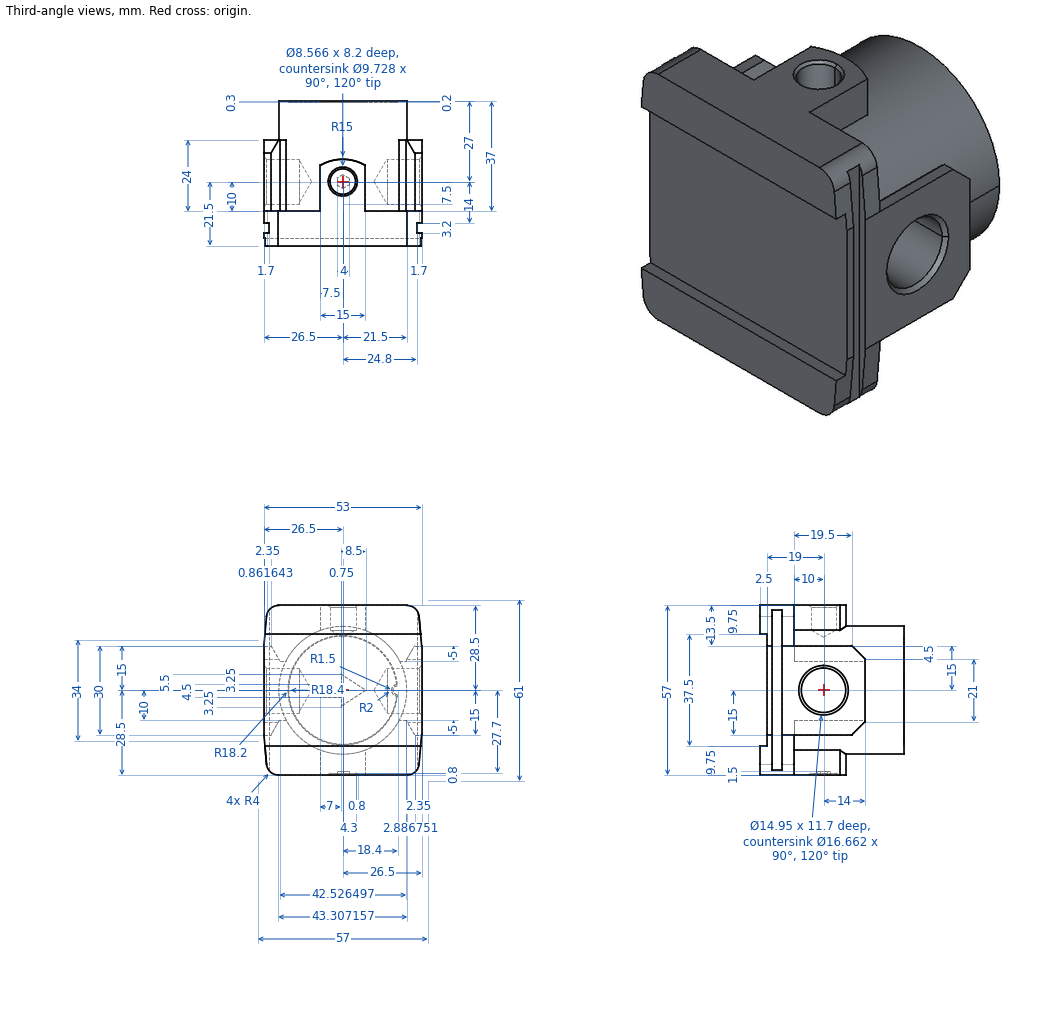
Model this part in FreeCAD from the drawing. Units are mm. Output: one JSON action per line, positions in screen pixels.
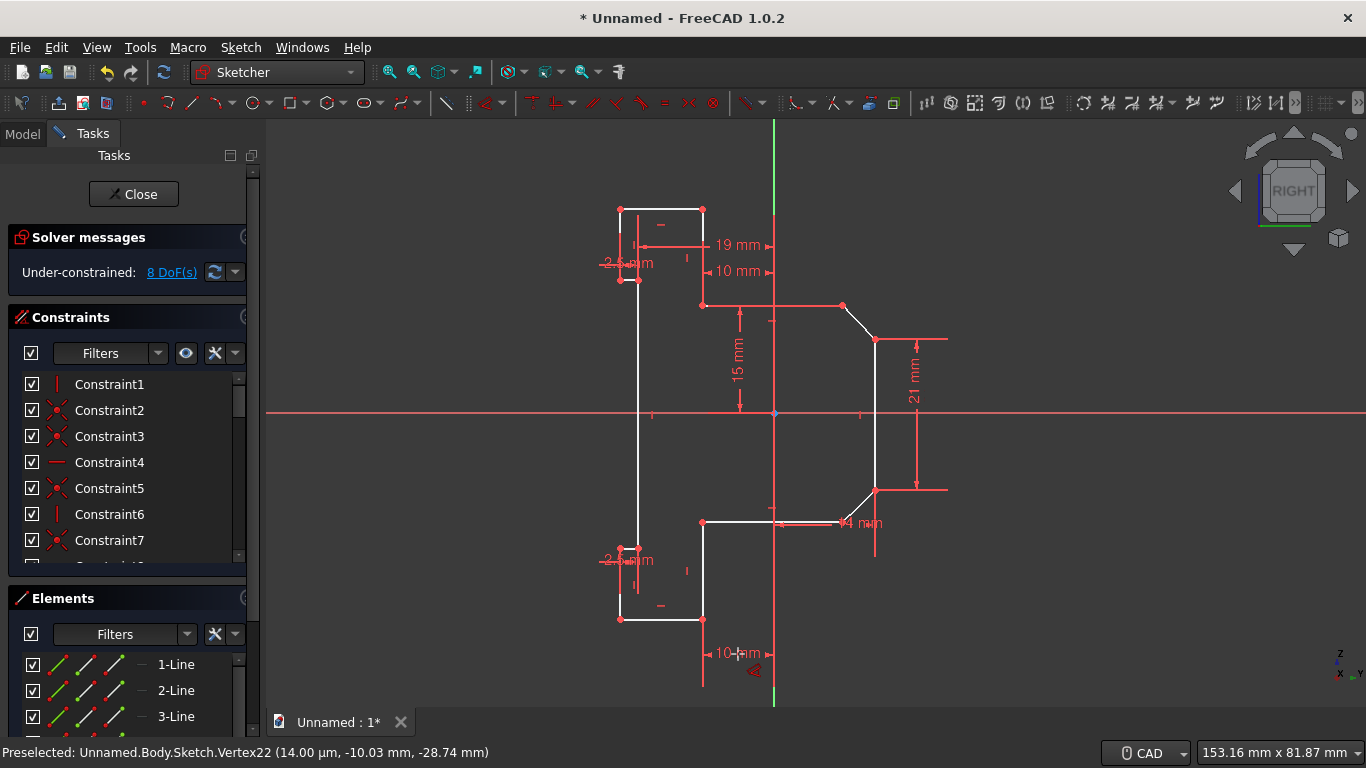
{"action": "left_click", "coordinate": [703, 522]}
{"action": "left_click", "coordinate": [669, 468]}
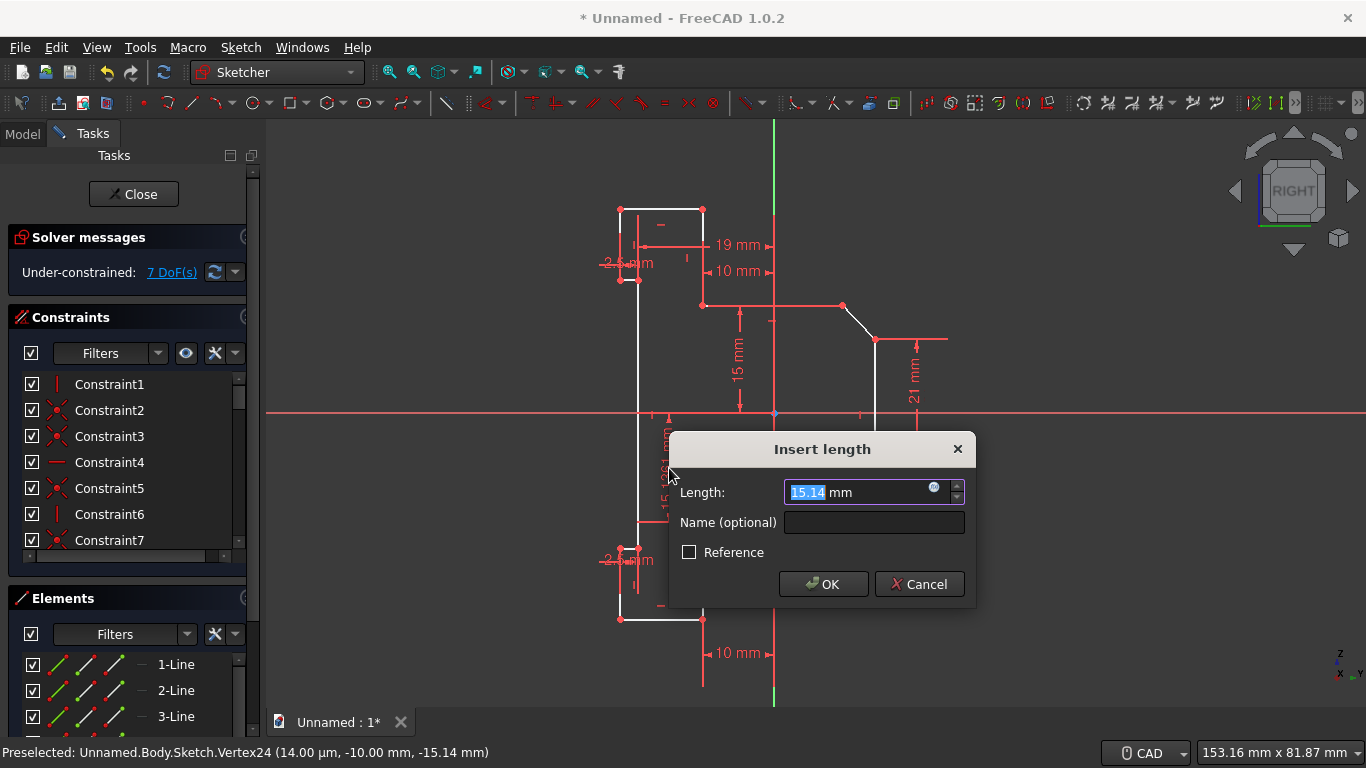
{"action": "type", "text": "15"}
{"action": "key", "text": "Return"}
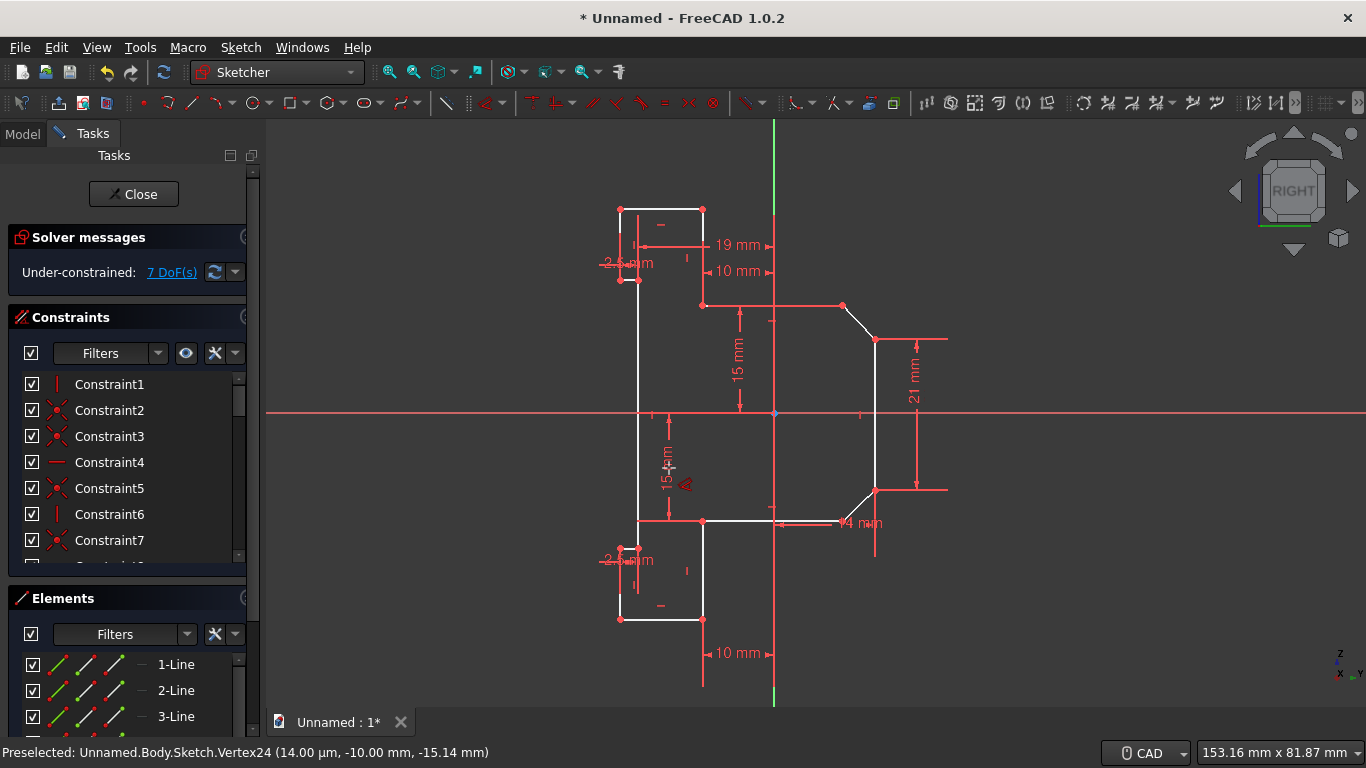
{"action": "left_click", "coordinate": [801, 306]}
{"action": "left_click", "coordinate": [822, 272]}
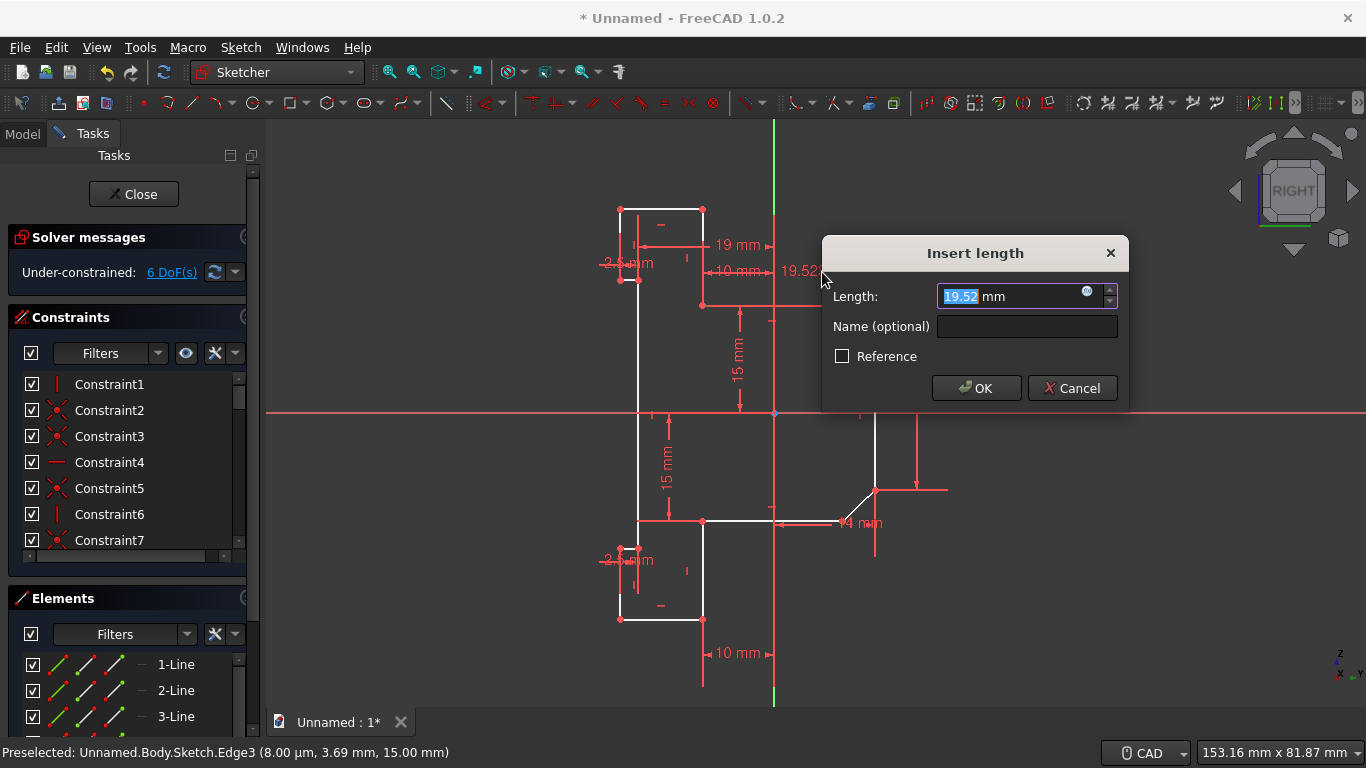
{"action": "type", "text": "19.5"}
{"action": "key", "text": "Return"}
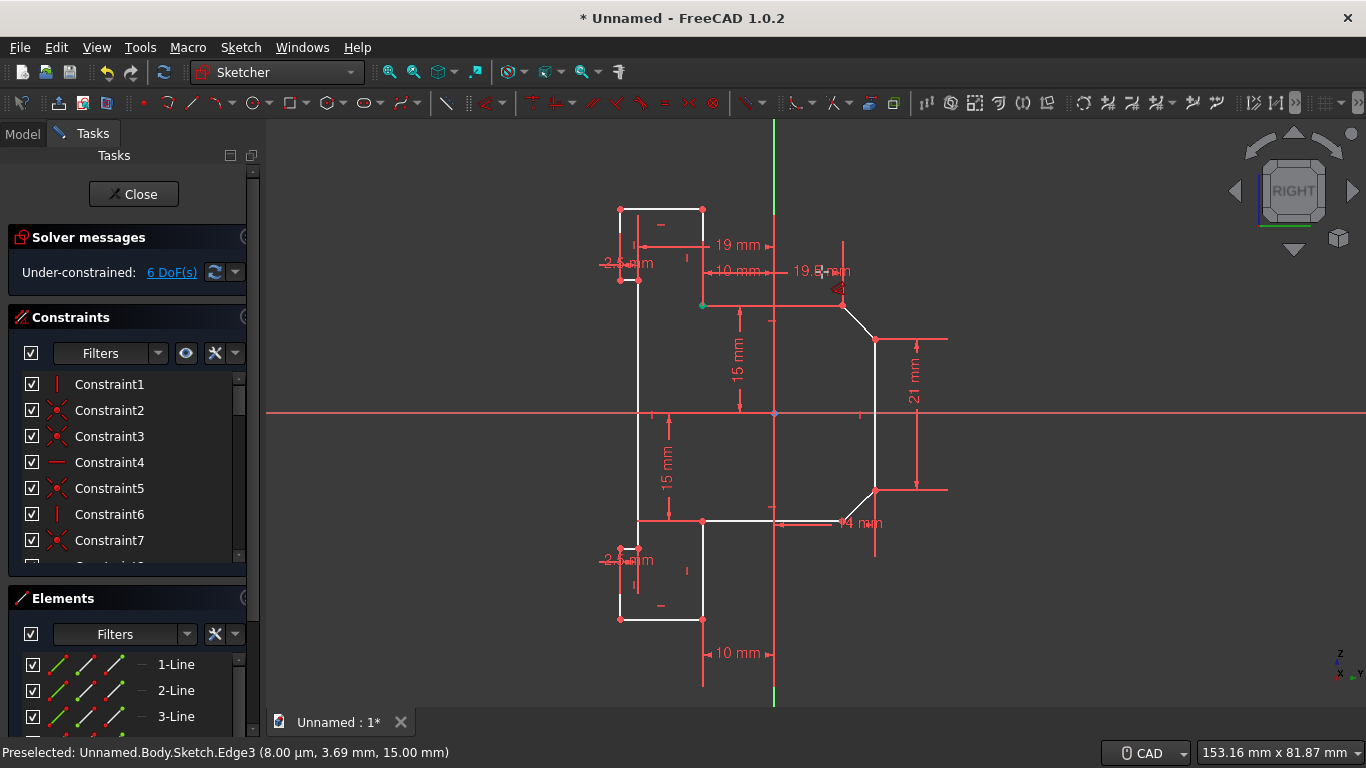
{"action": "left_click", "coordinate": [703, 277]}
{"action": "left_click", "coordinate": [669, 224]}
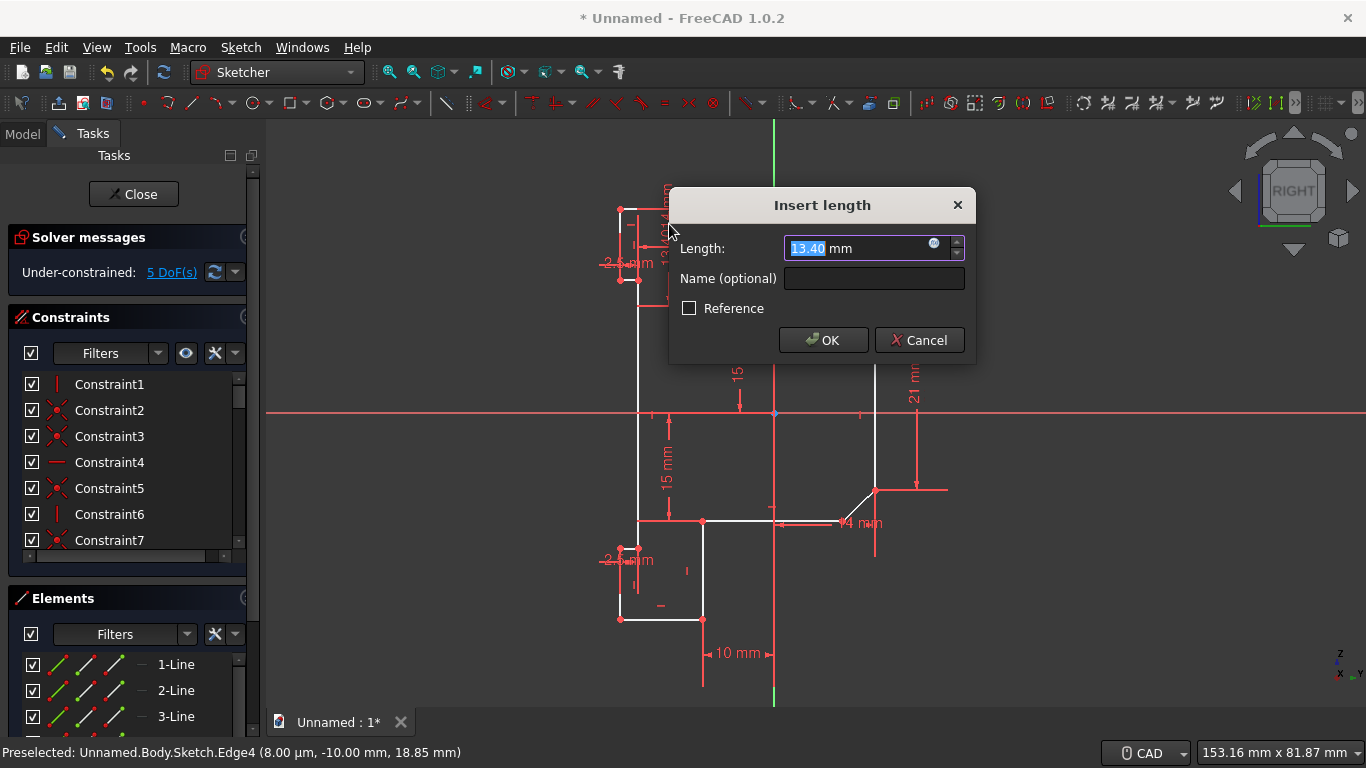
{"action": "type", "text": "13.5"}
{"action": "key", "text": "Return"}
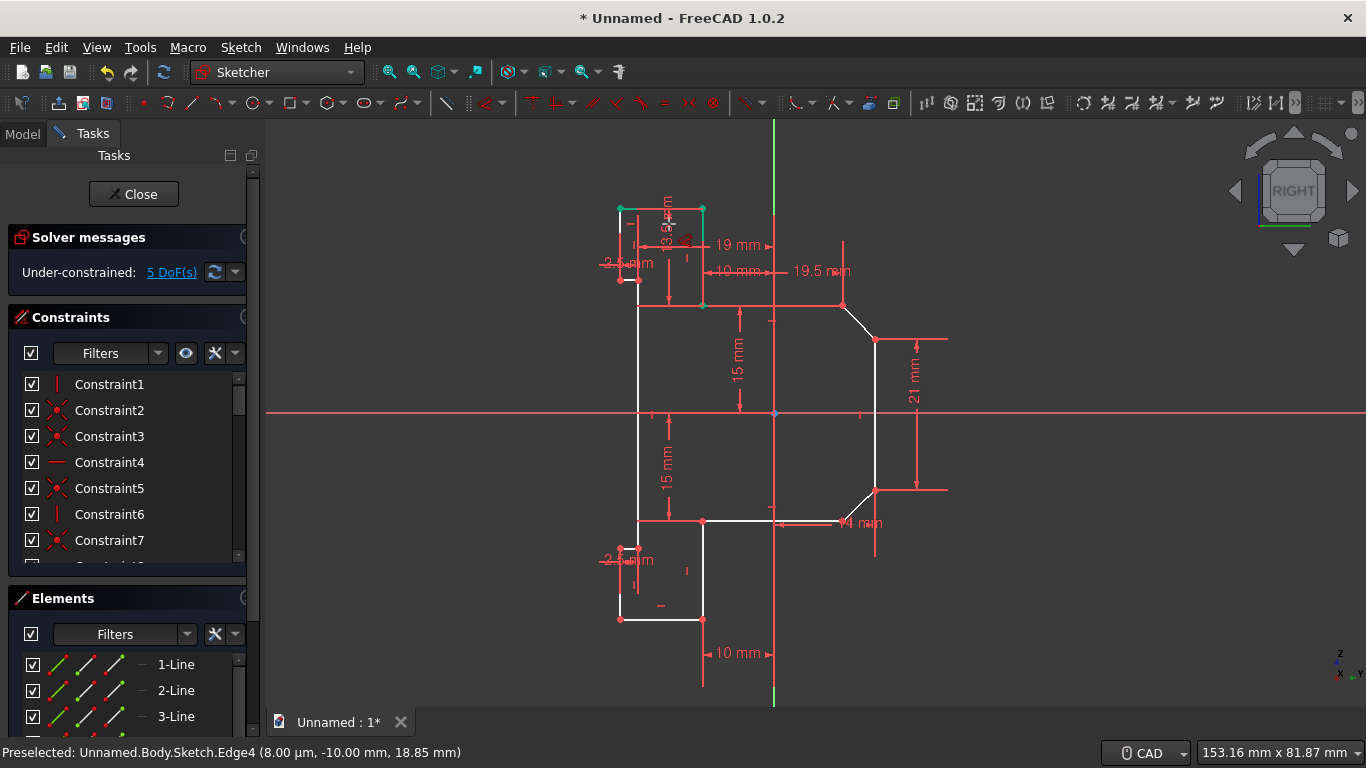
{"action": "left_click", "coordinate": [620, 230]}
{"action": "left_click", "coordinate": [586, 244]}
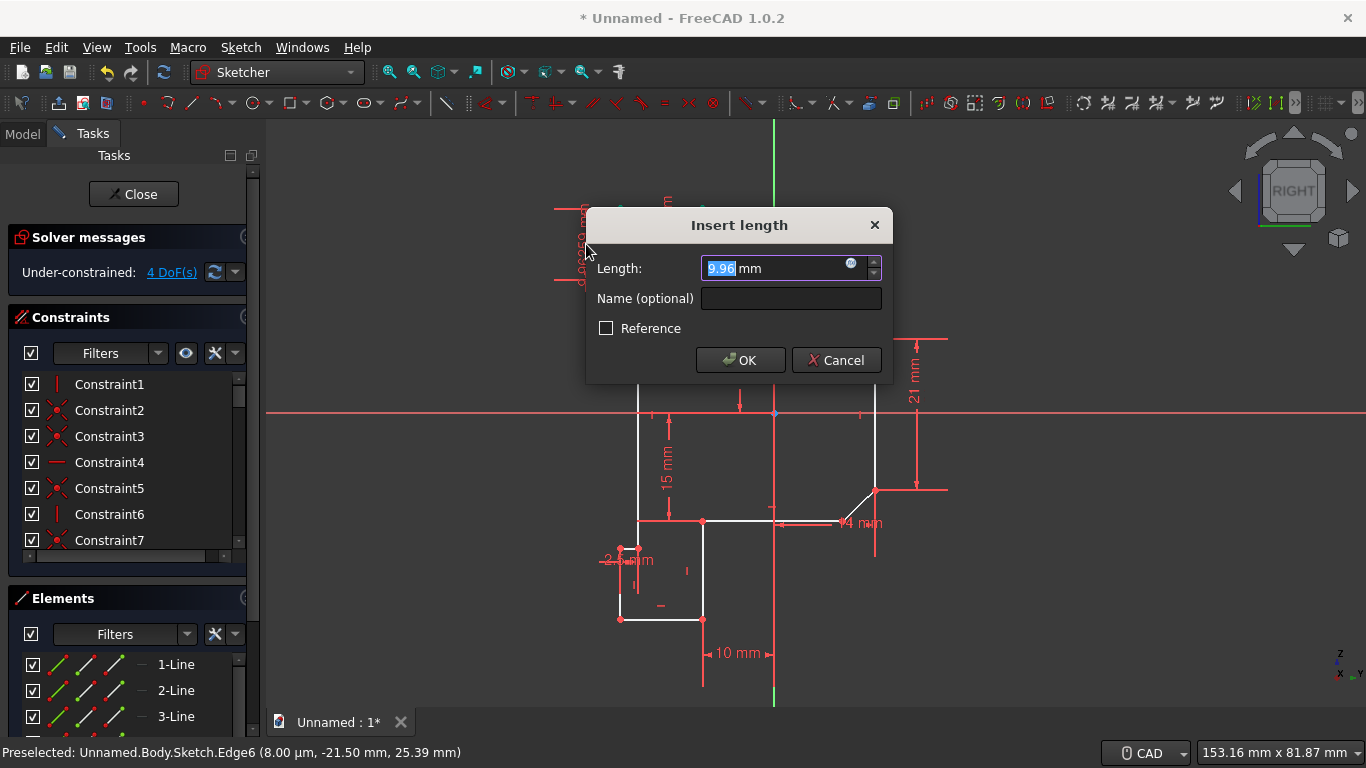
{"action": "type", "text": "9.75"}
{"action": "key", "text": "Return"}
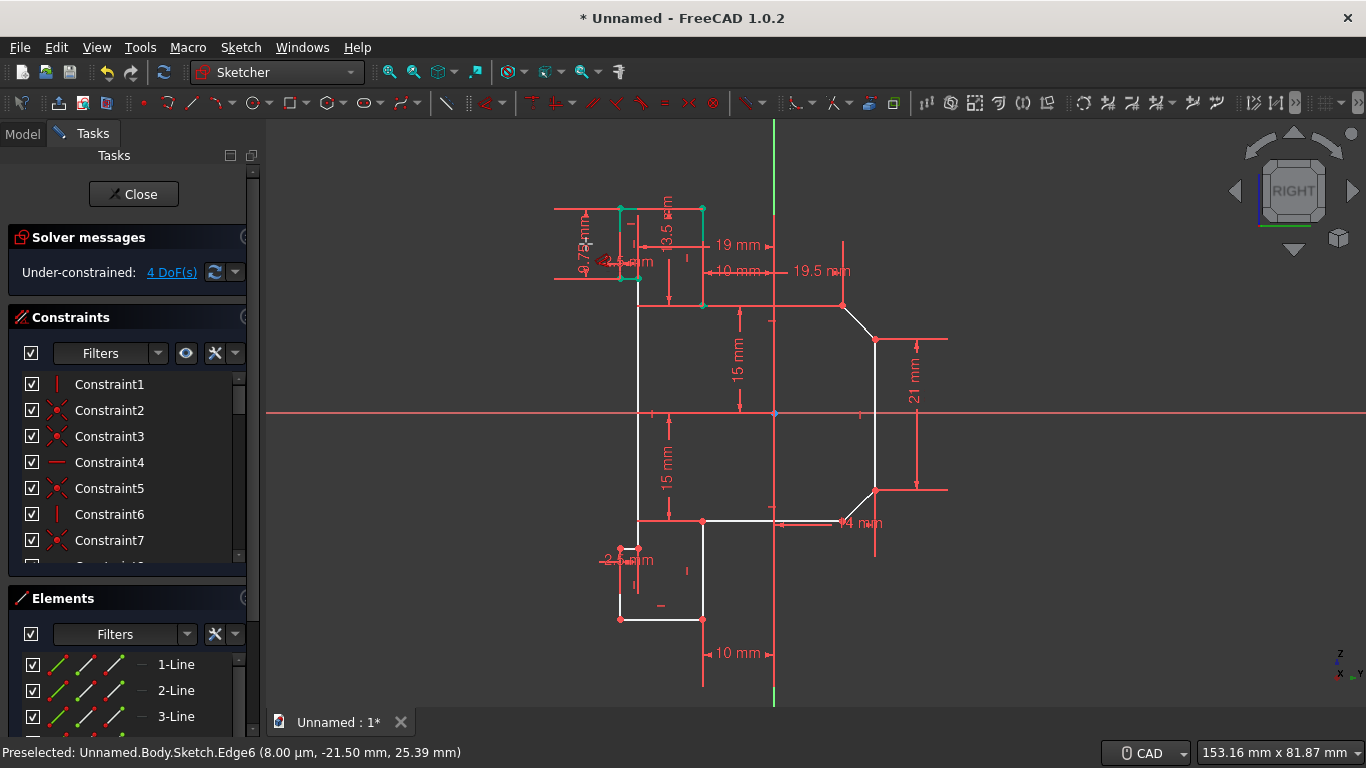
{"action": "left_click", "coordinate": [638, 360]}
{"action": "left_click", "coordinate": [604, 352]}